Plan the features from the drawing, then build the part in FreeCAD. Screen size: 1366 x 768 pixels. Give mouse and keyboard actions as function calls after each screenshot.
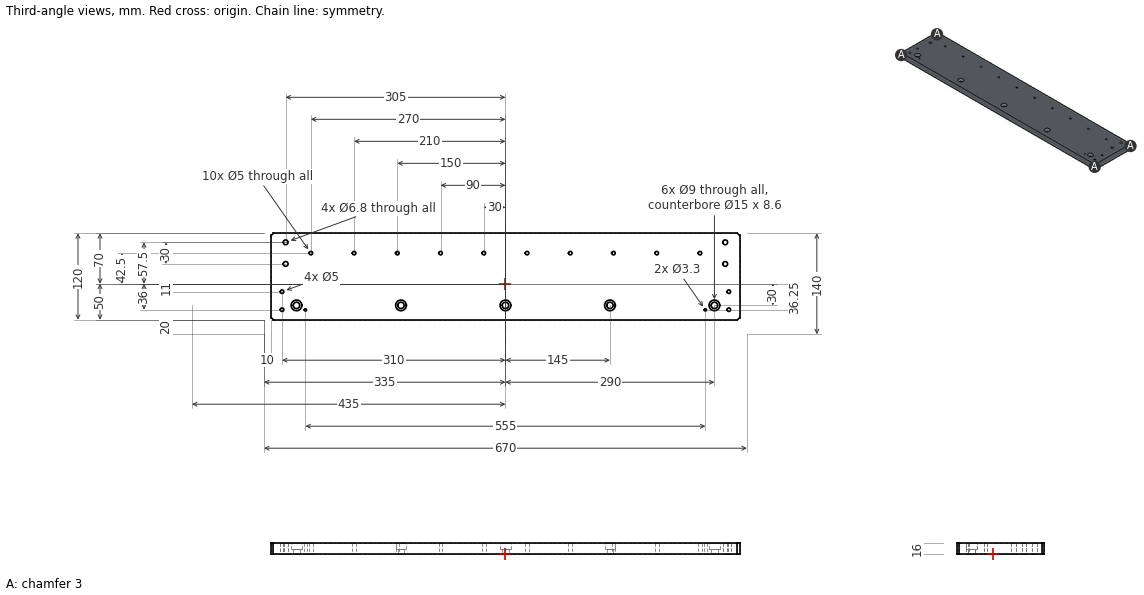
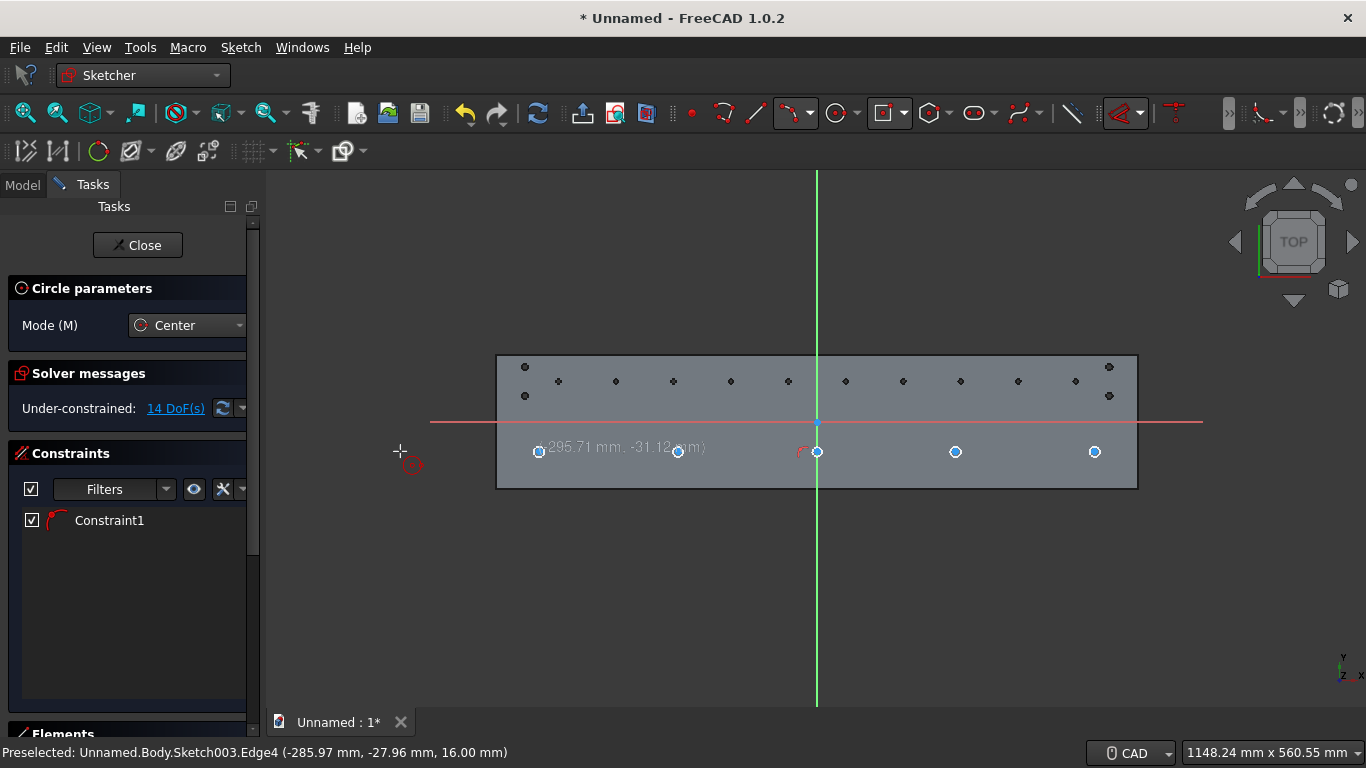
click(400, 451)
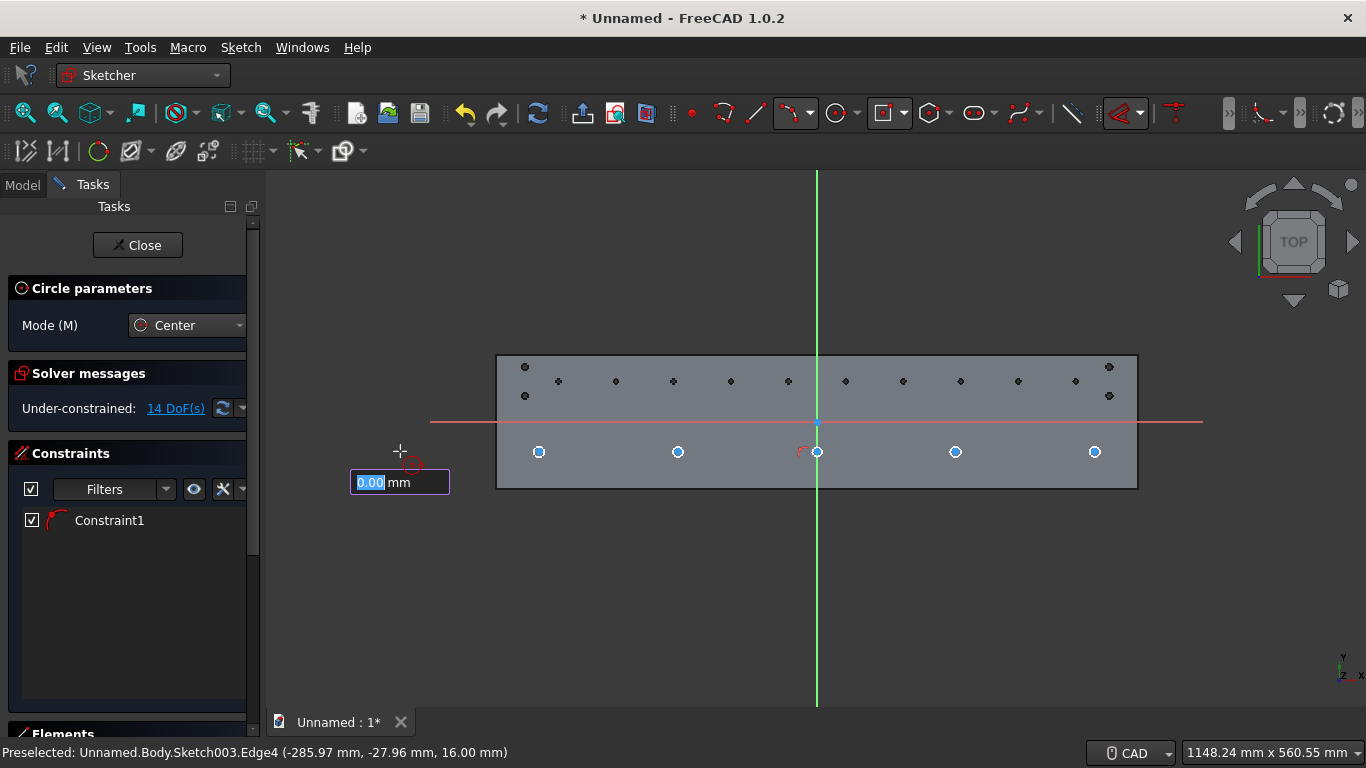
scroll(403, 448, up, 7)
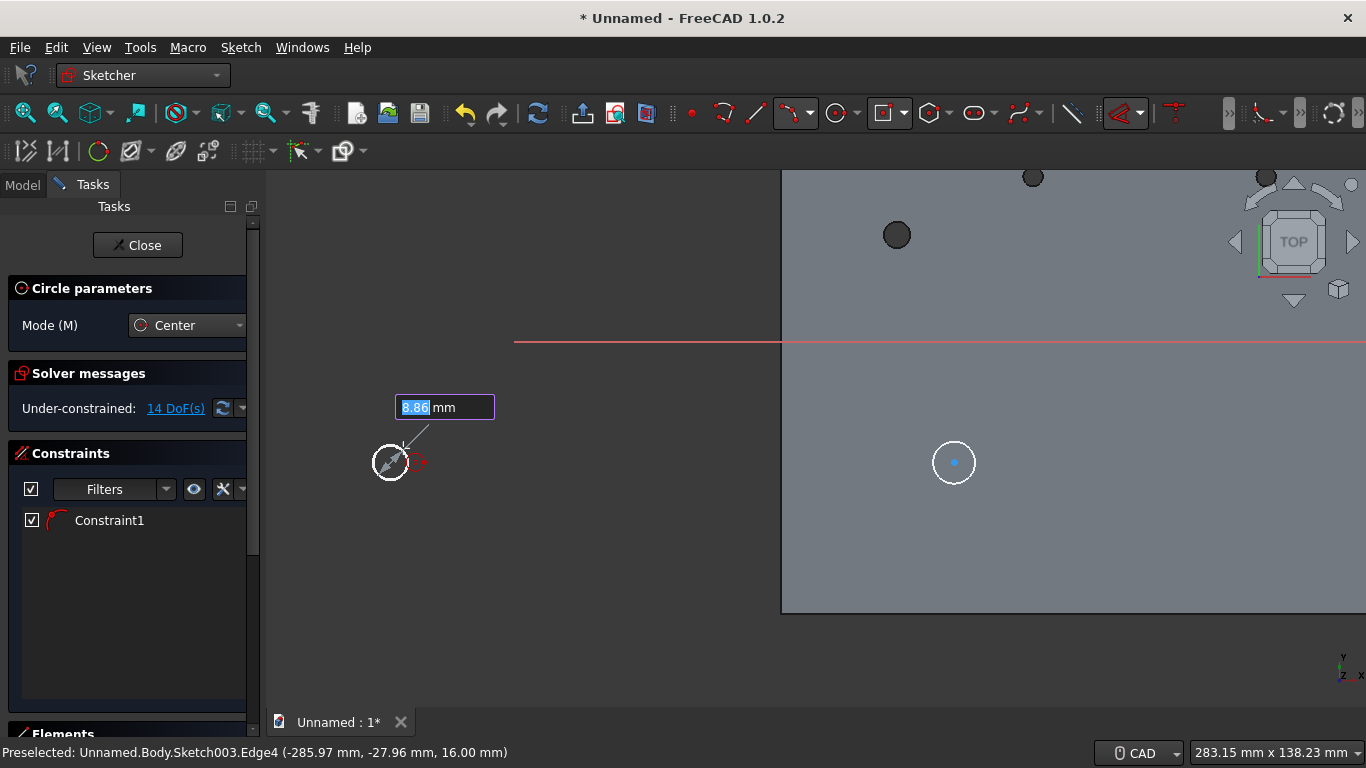
click(404, 446)
key(Escape)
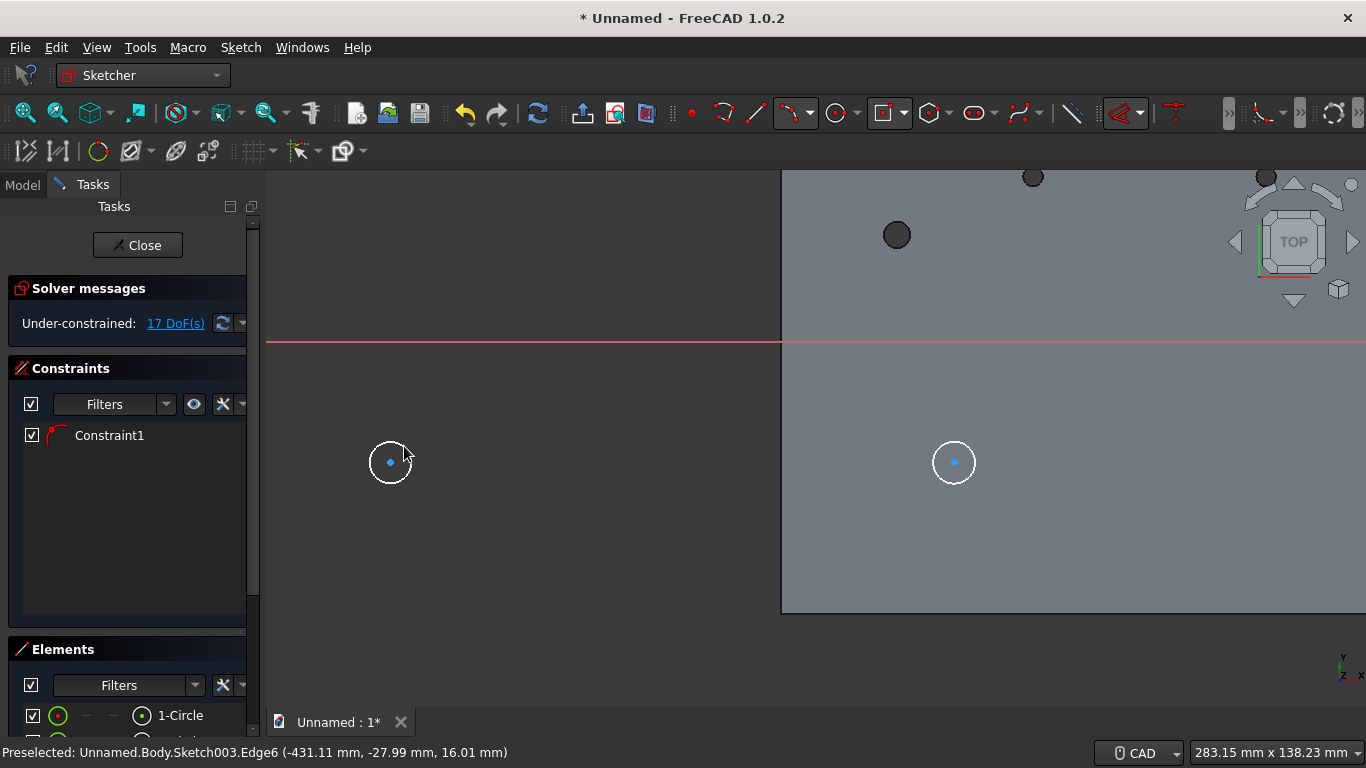
scroll(403, 448, down, 7)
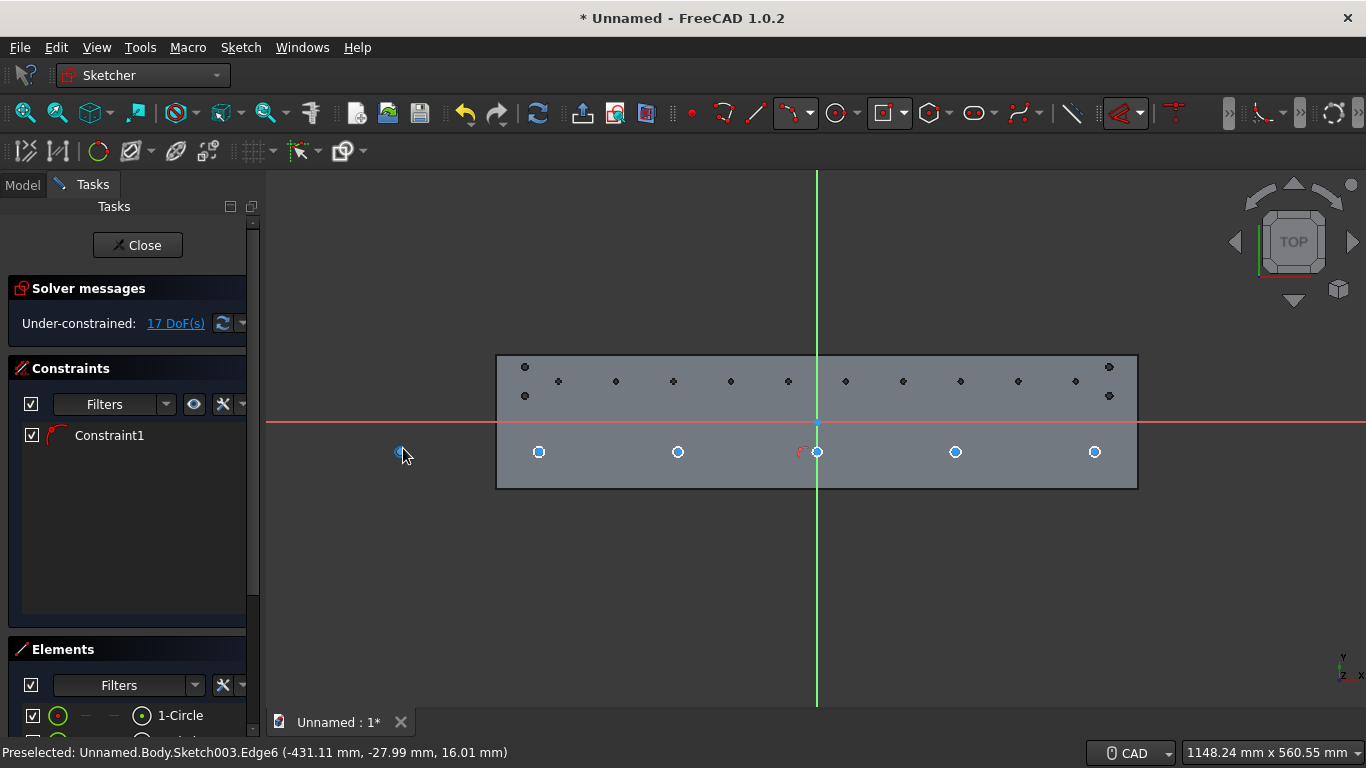
scroll(1098, 448, up, 5)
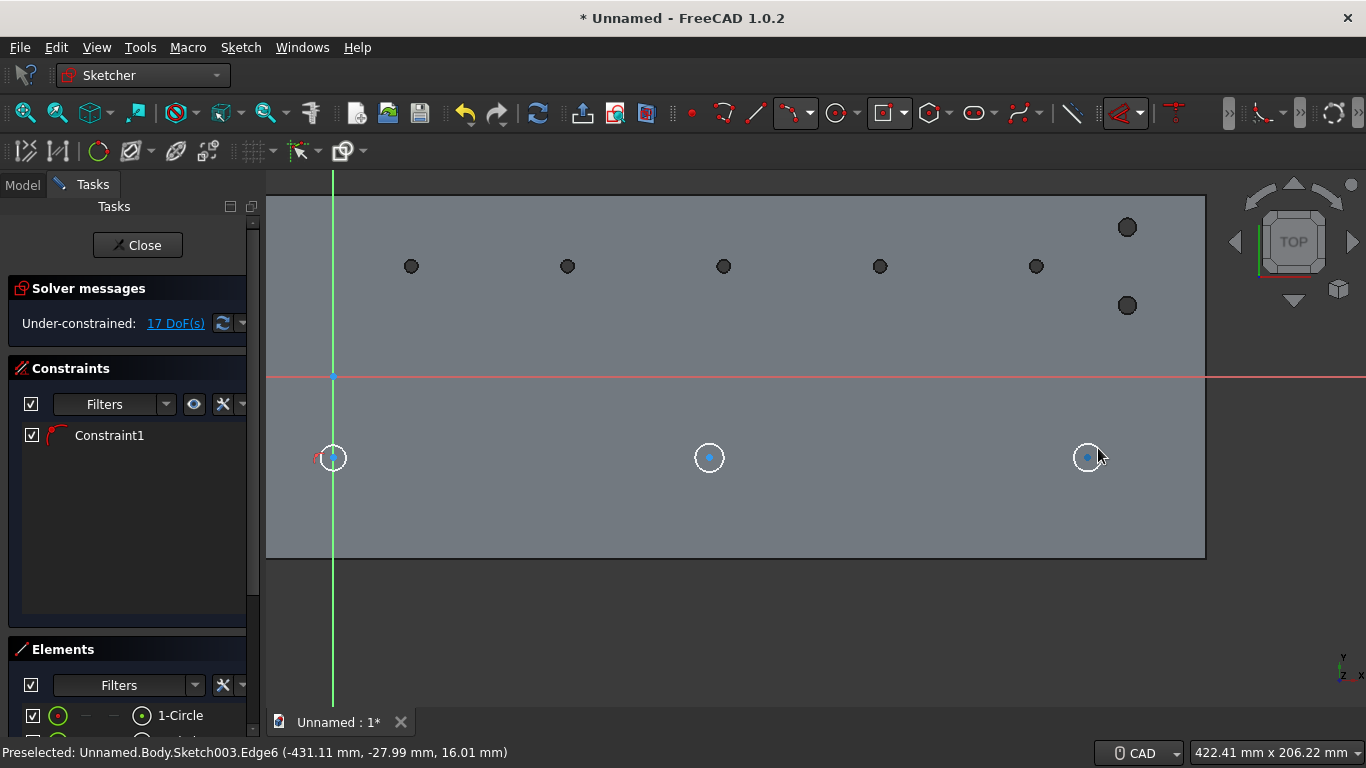
click(1098, 448)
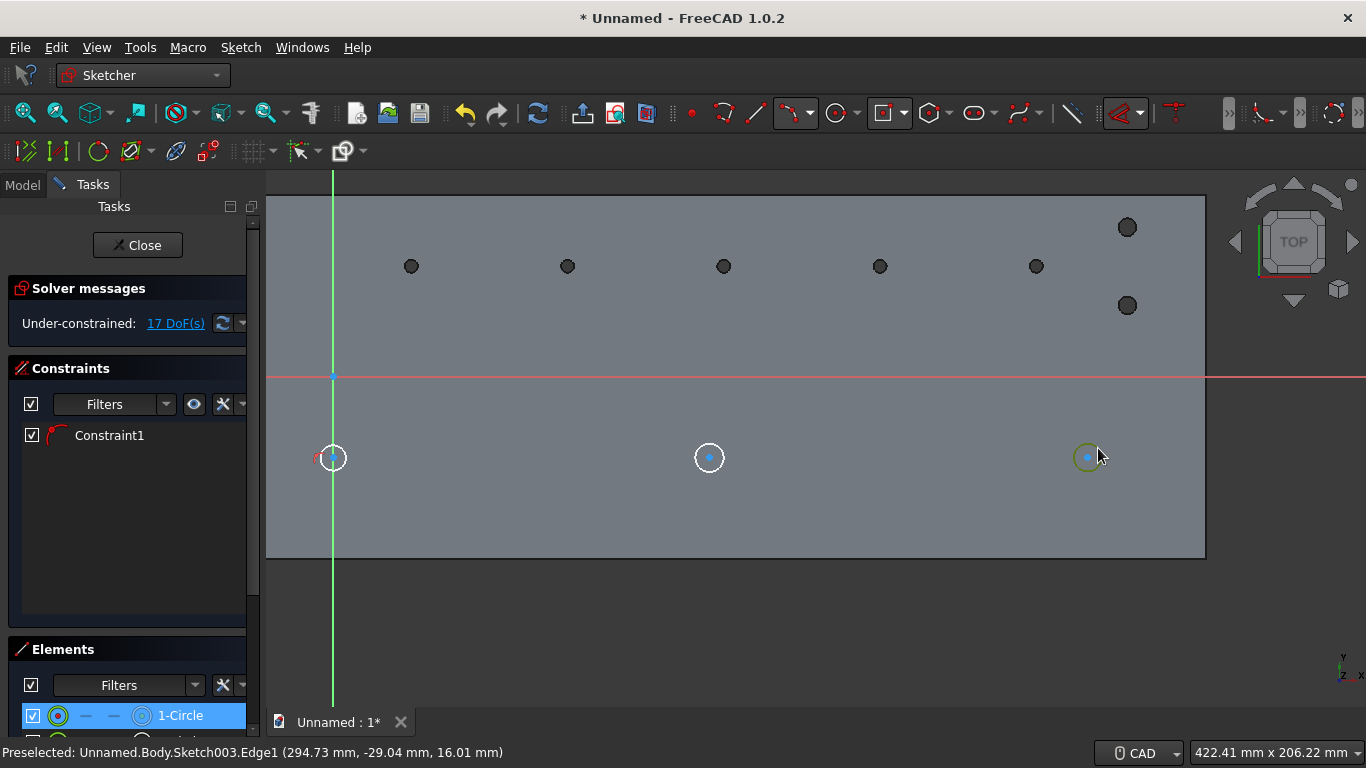
click(720, 448)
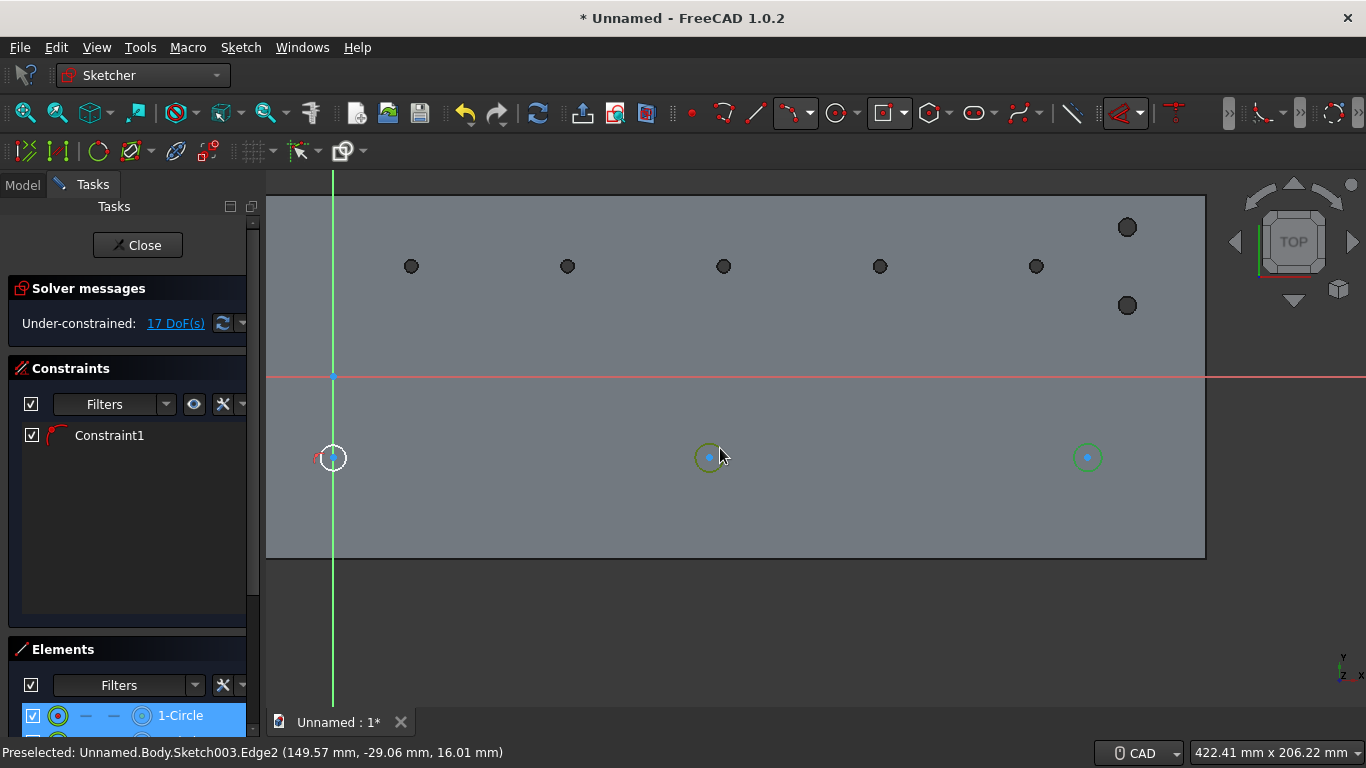
click(334, 445)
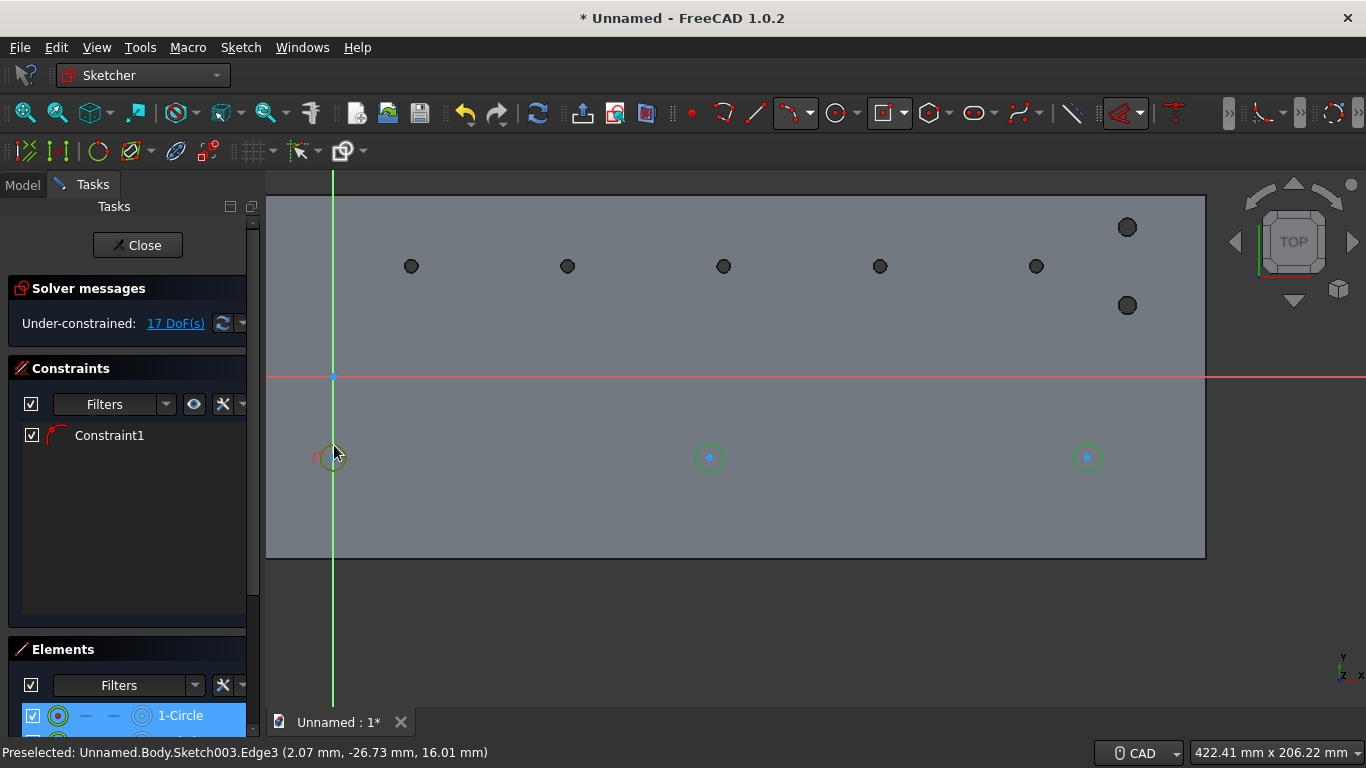
scroll(1098, 448, down, 5)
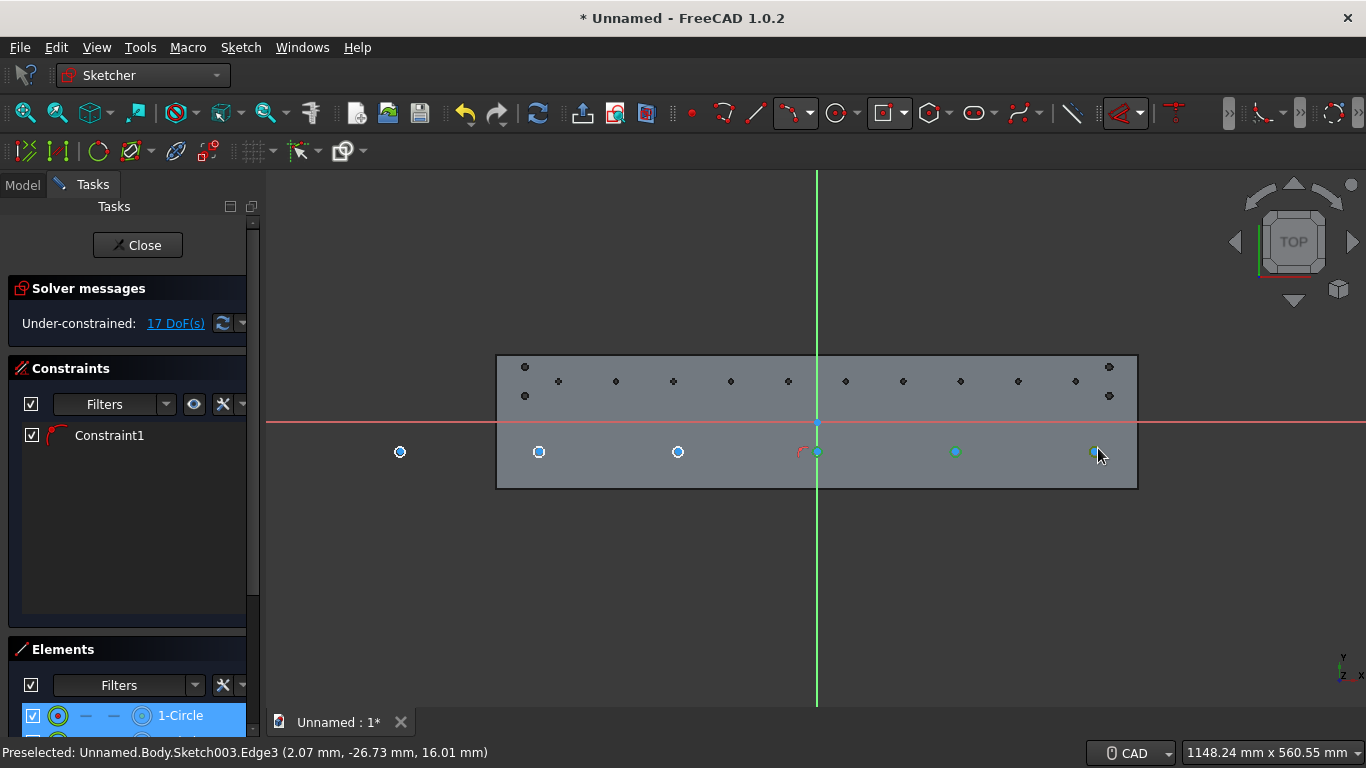
scroll(682, 448, up, 6)